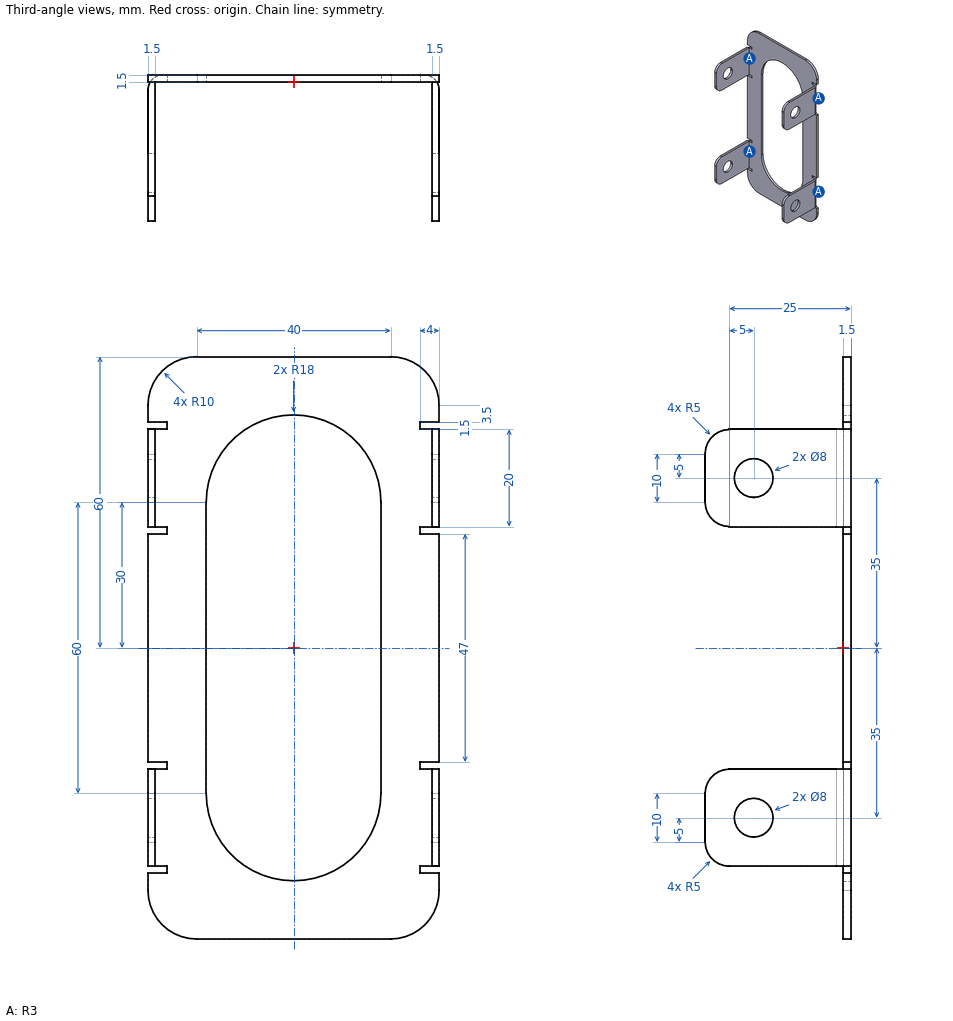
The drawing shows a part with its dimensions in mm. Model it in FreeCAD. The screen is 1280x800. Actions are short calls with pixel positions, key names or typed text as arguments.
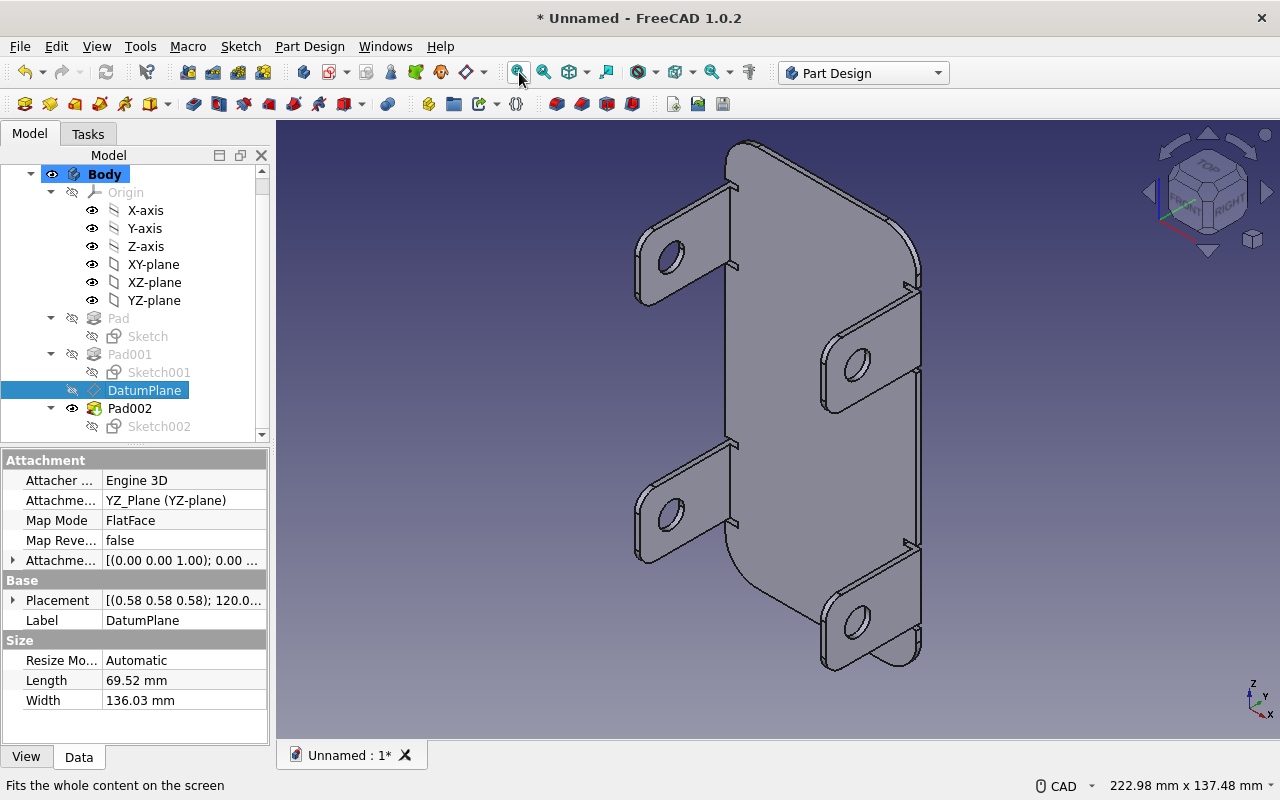
key(1)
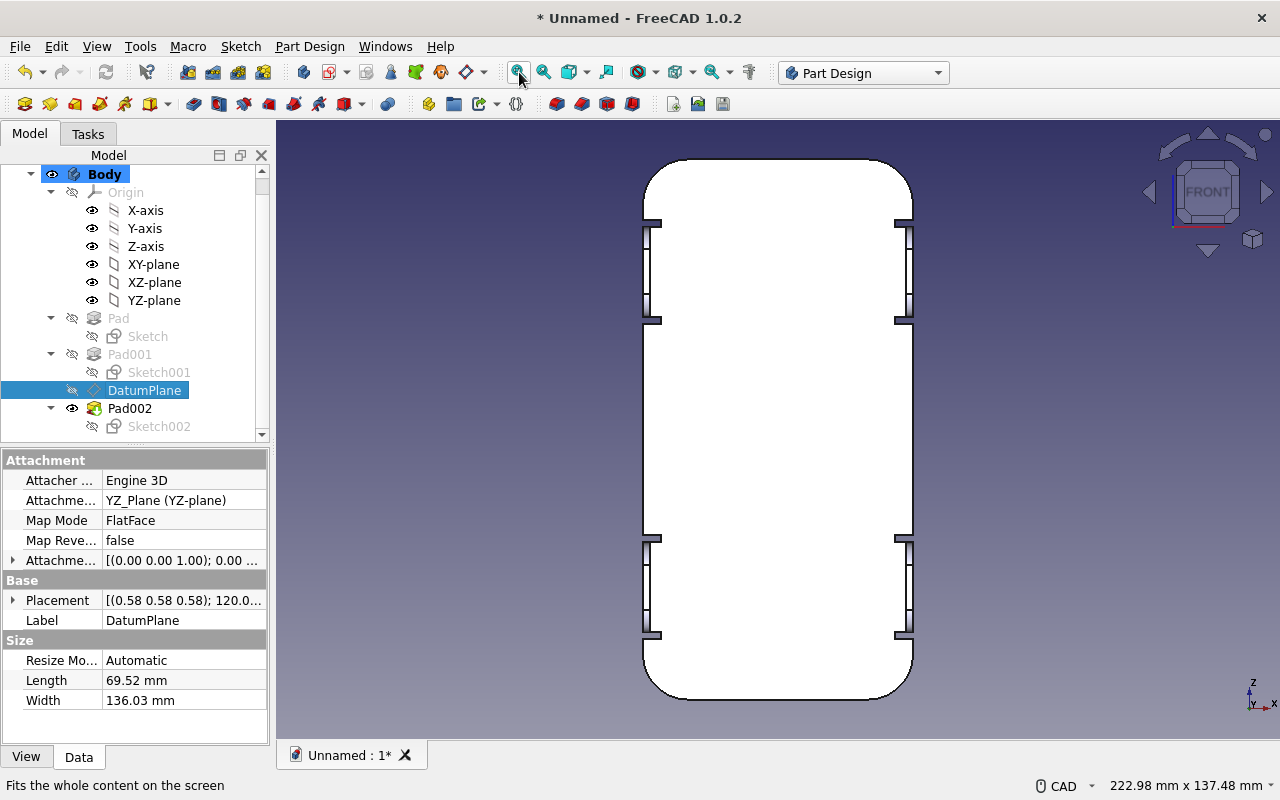
key(3)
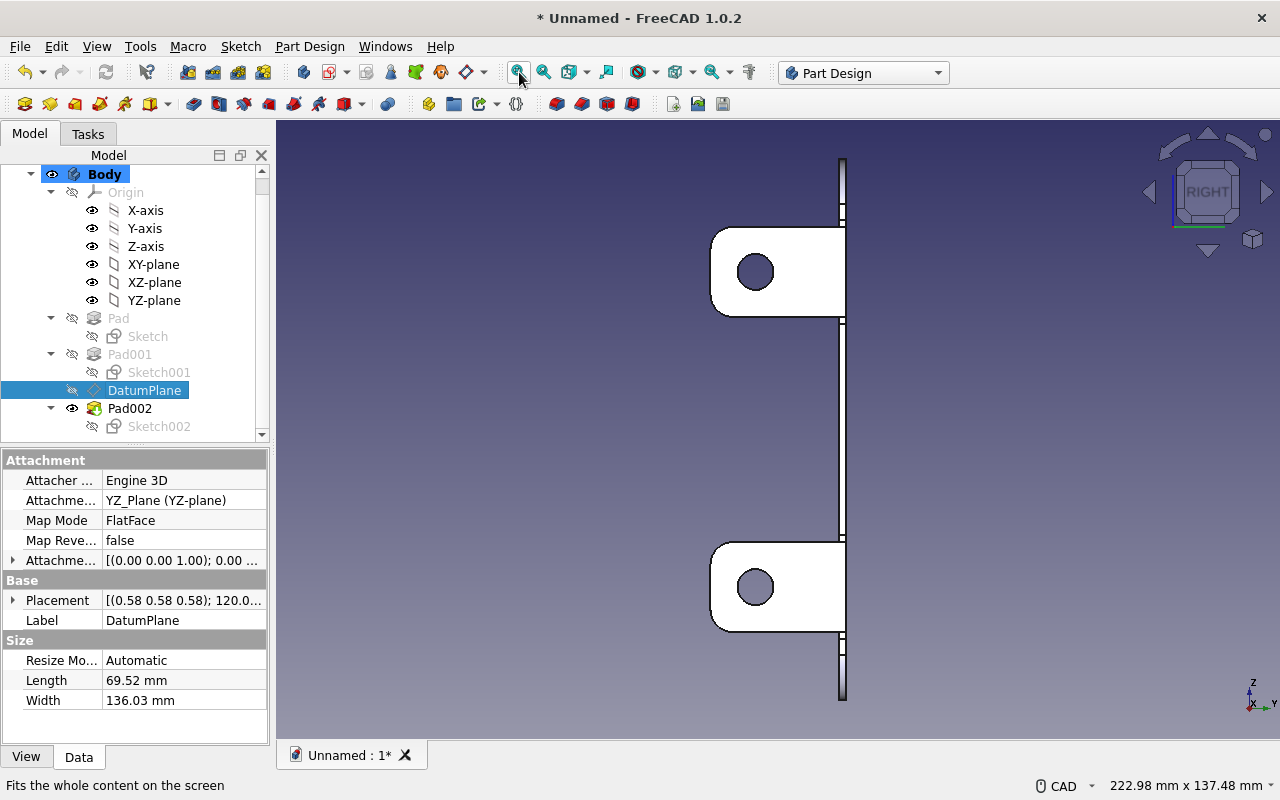
click(846, 271)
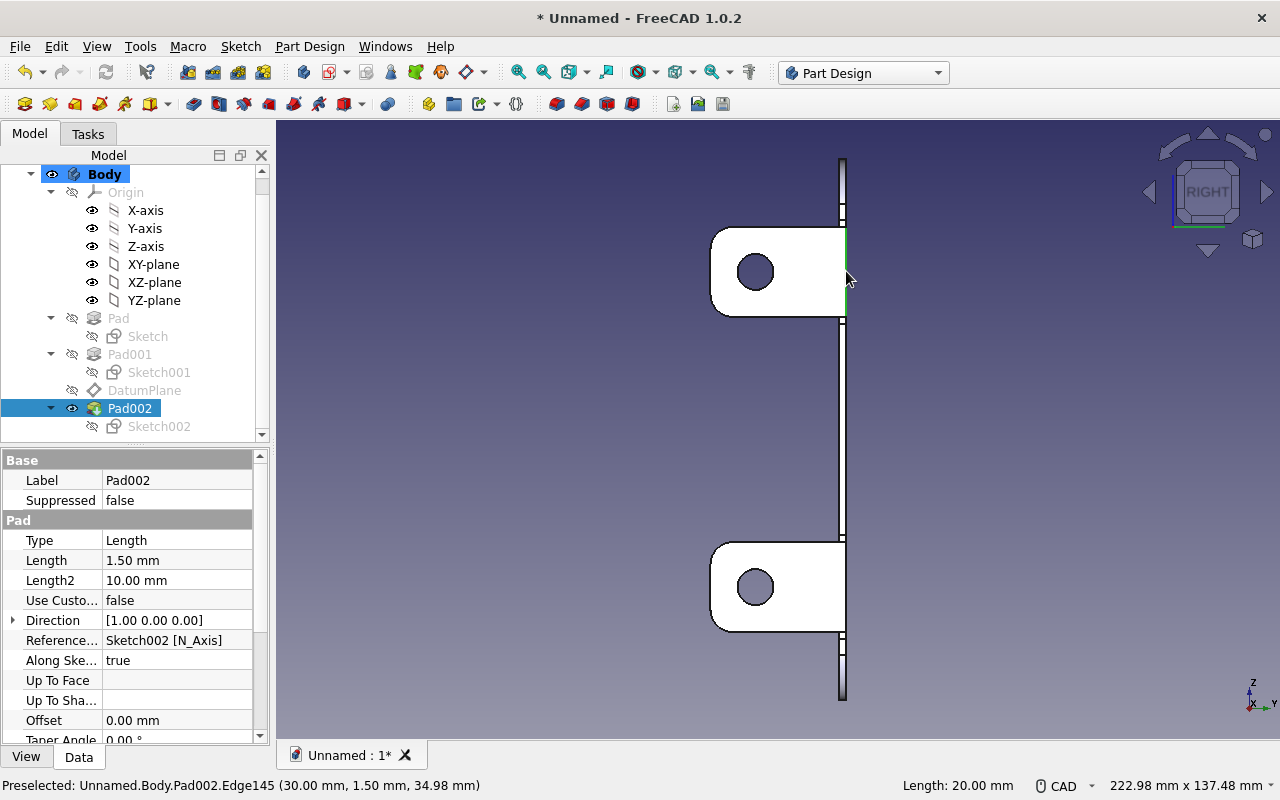
click(846, 586, ctrl)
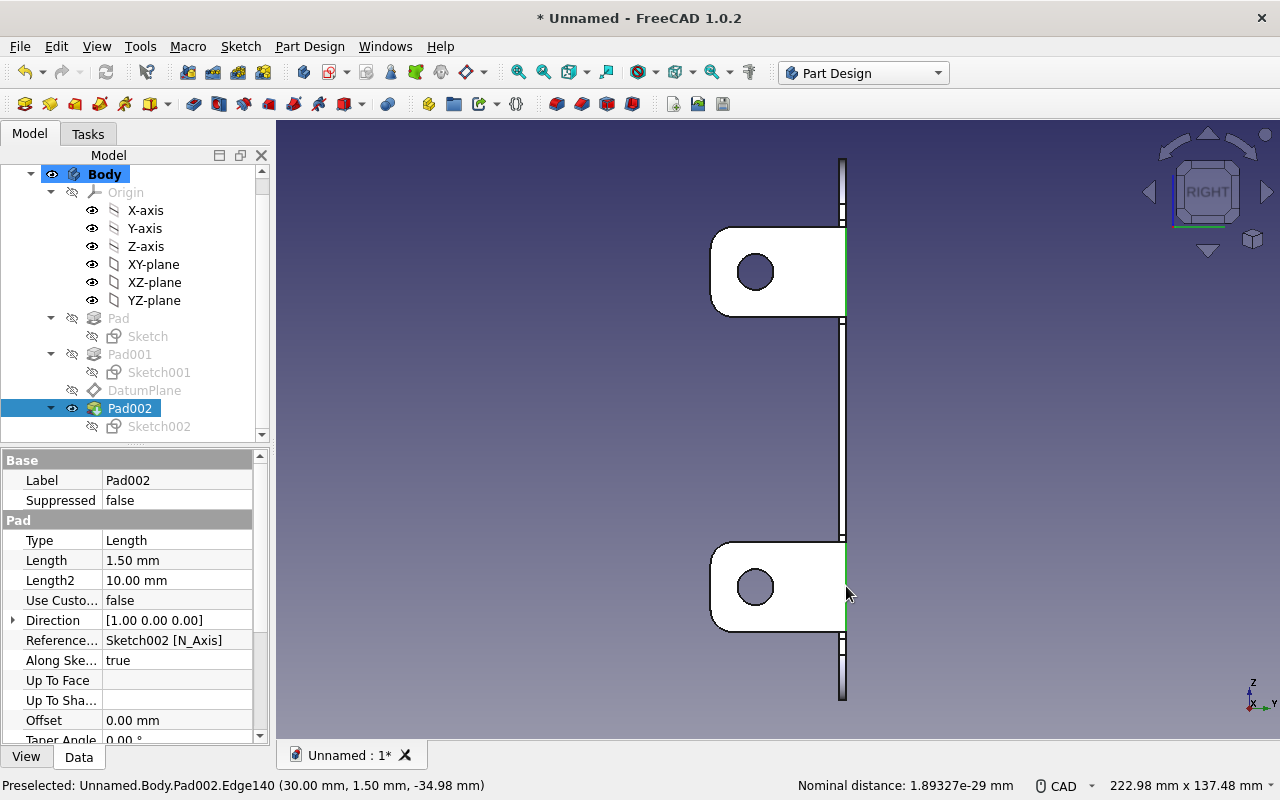
key(5)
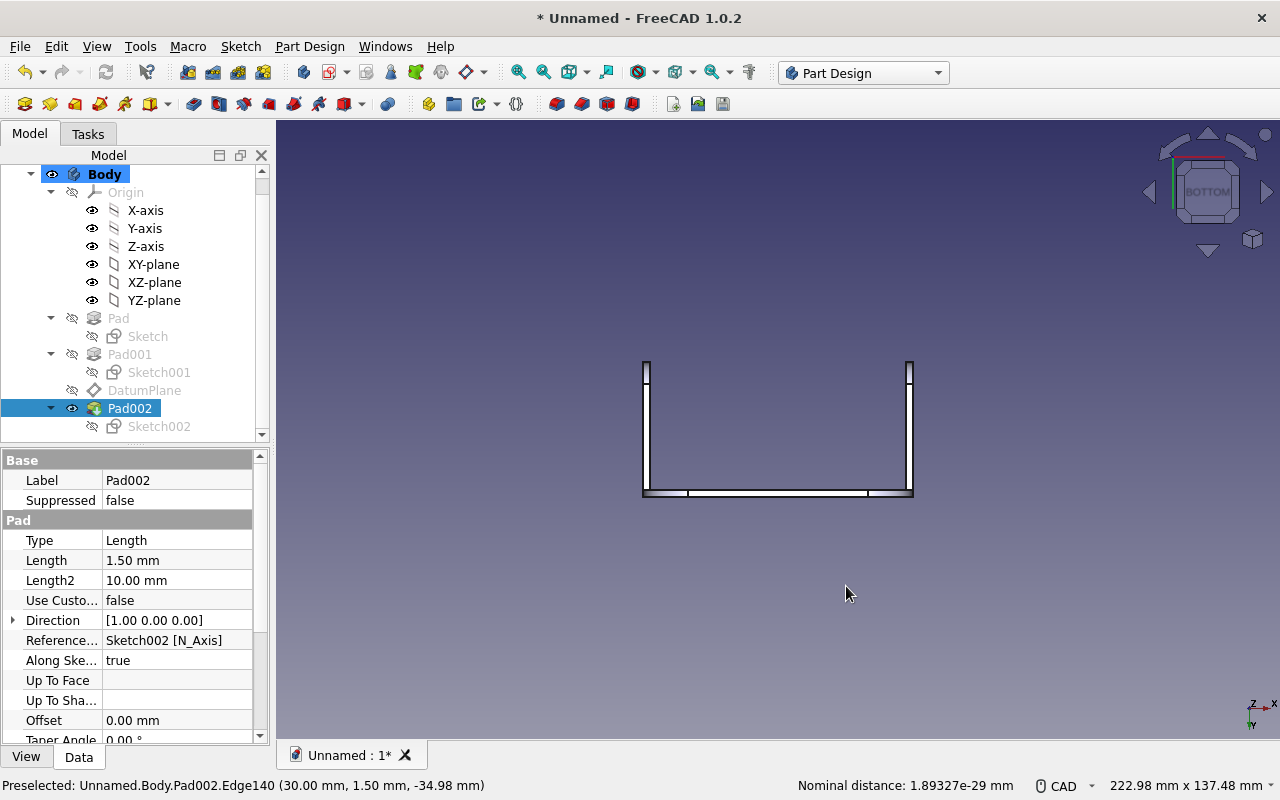
click(519, 72)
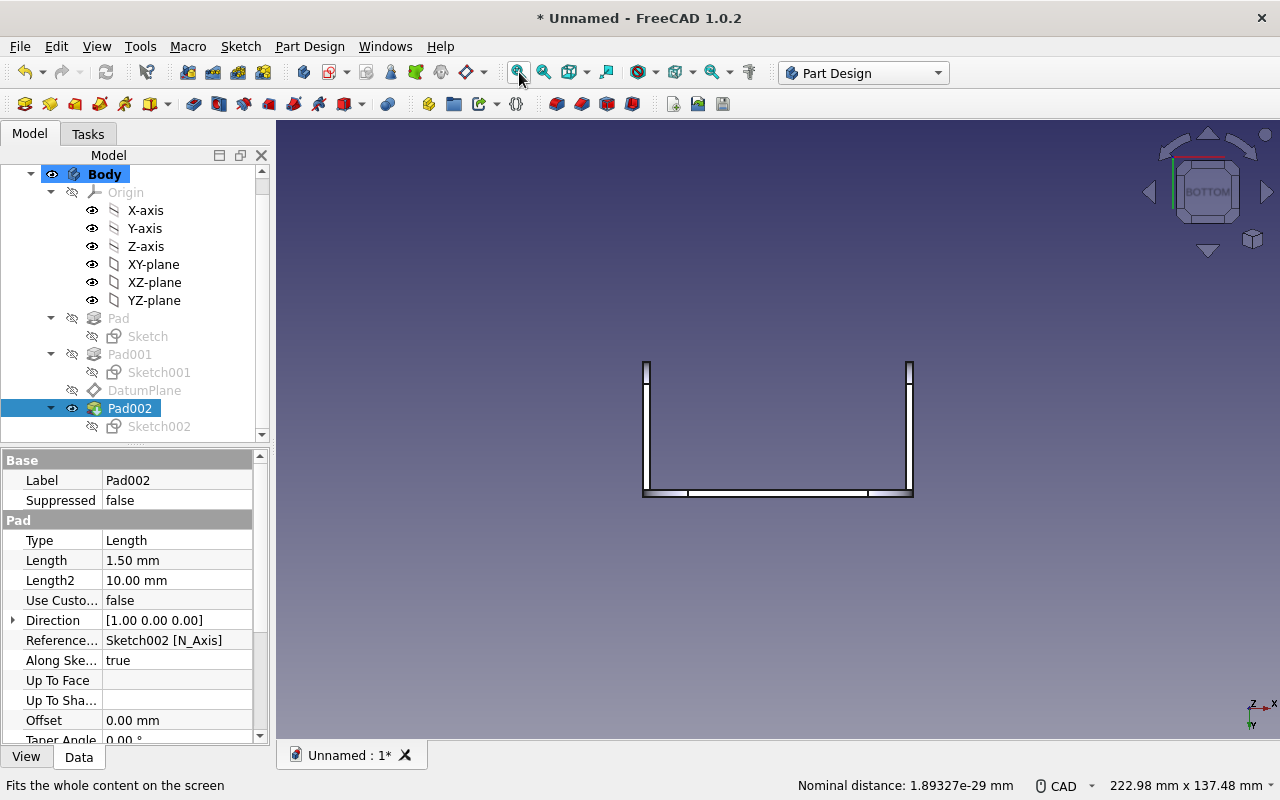
key(4)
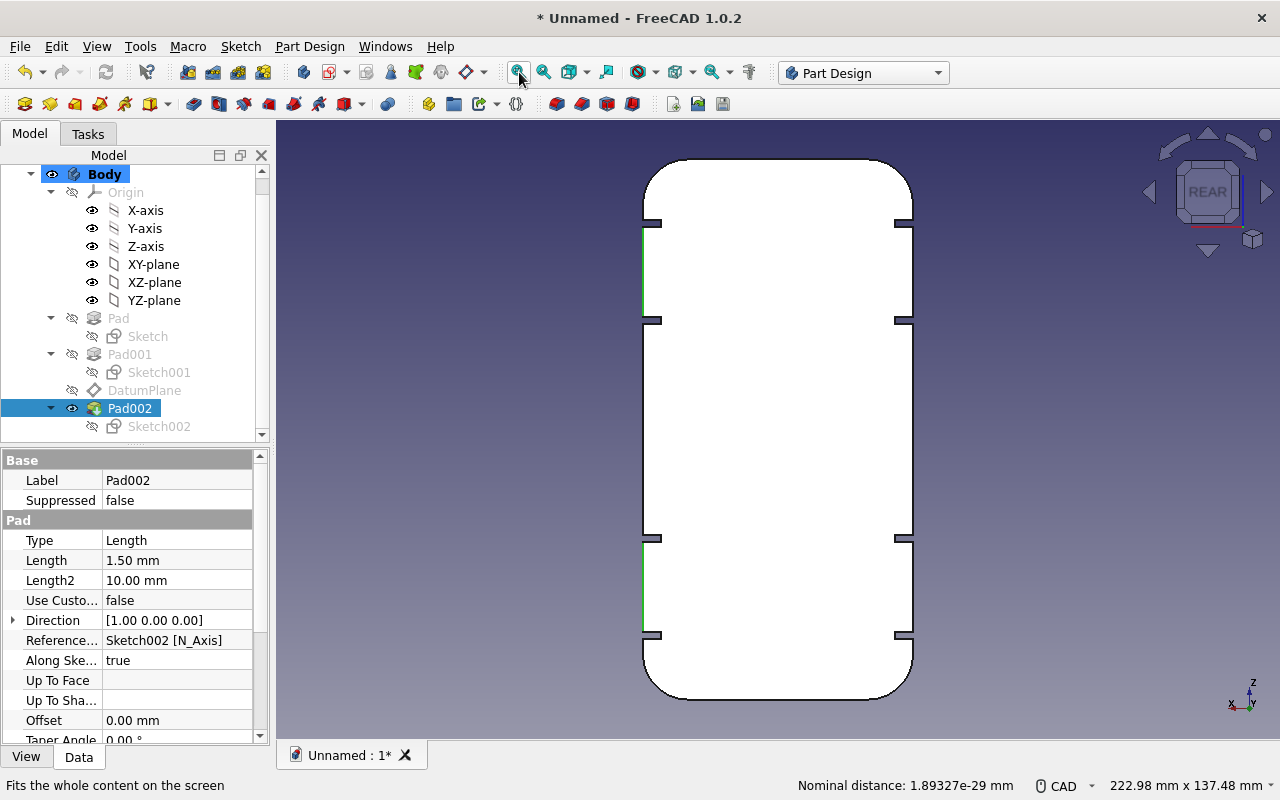
click(913, 586, ctrl)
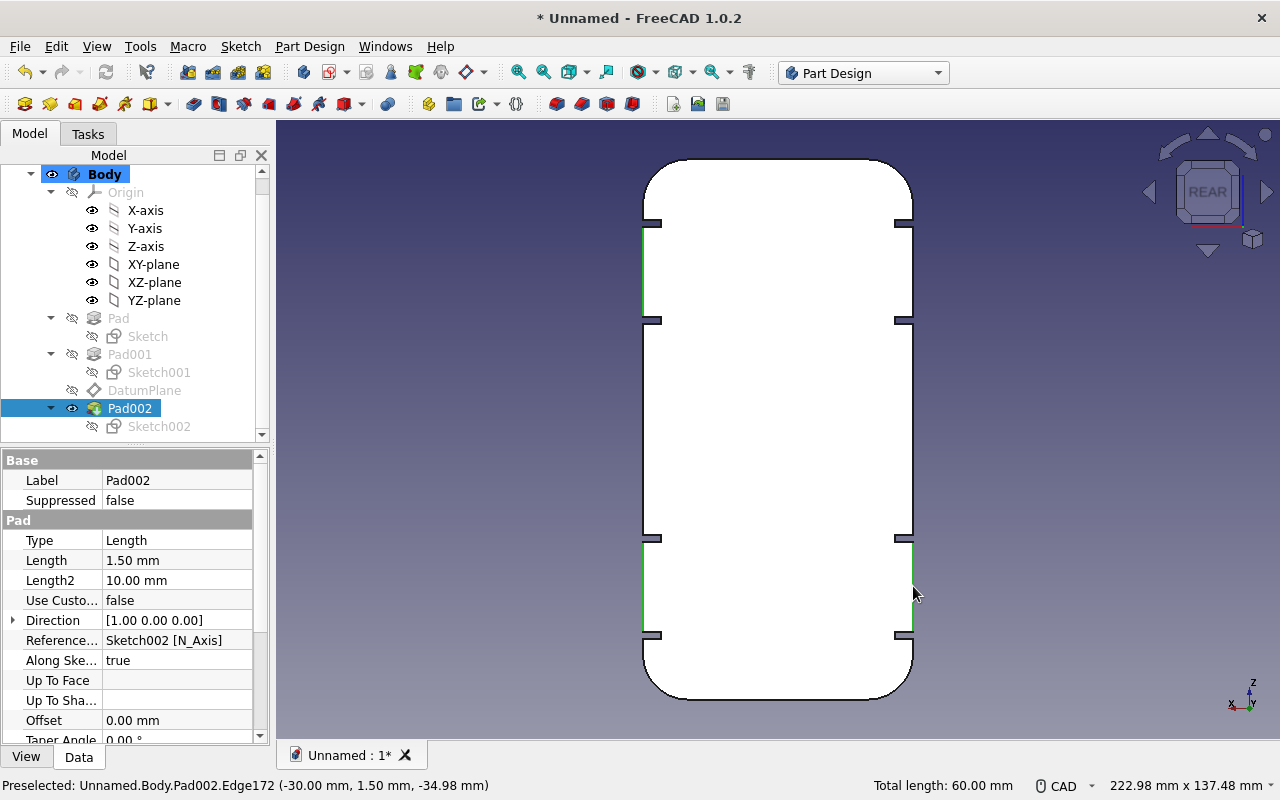
click(913, 271, ctrl)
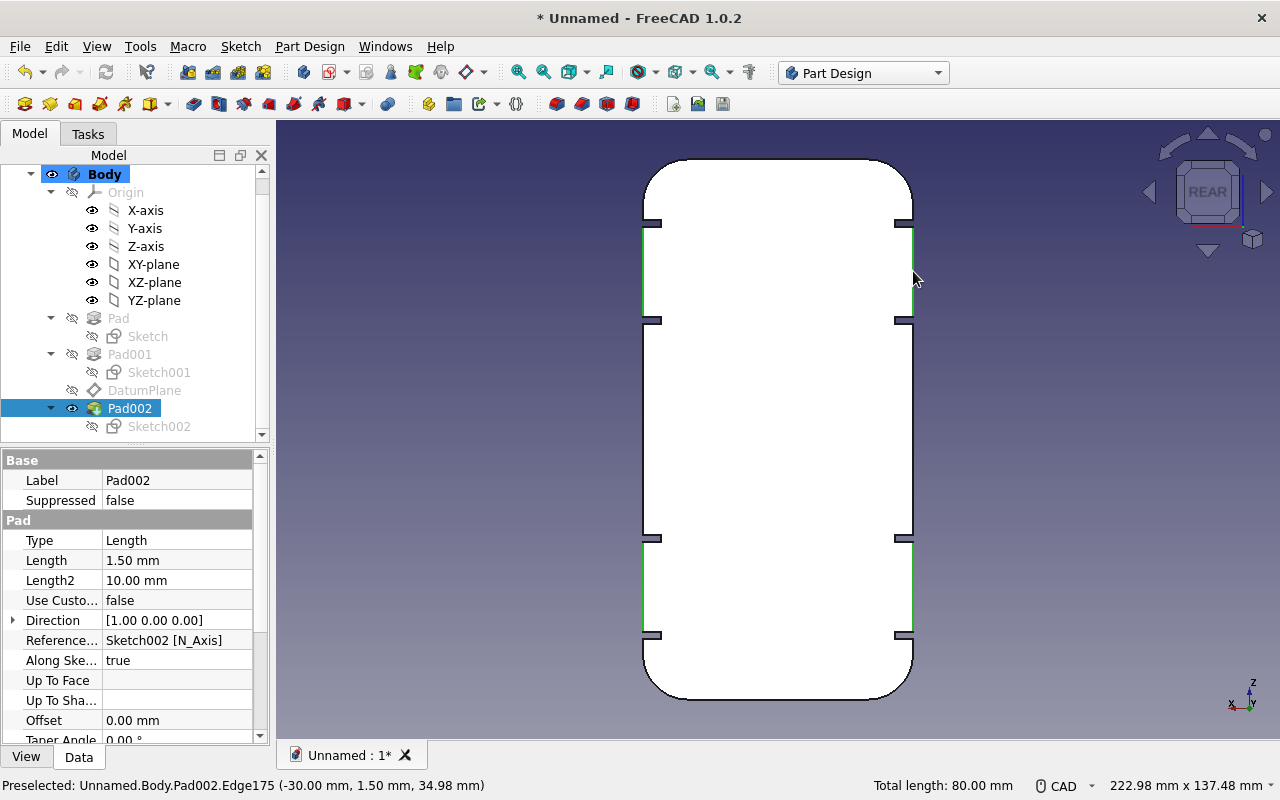
click(557, 104)